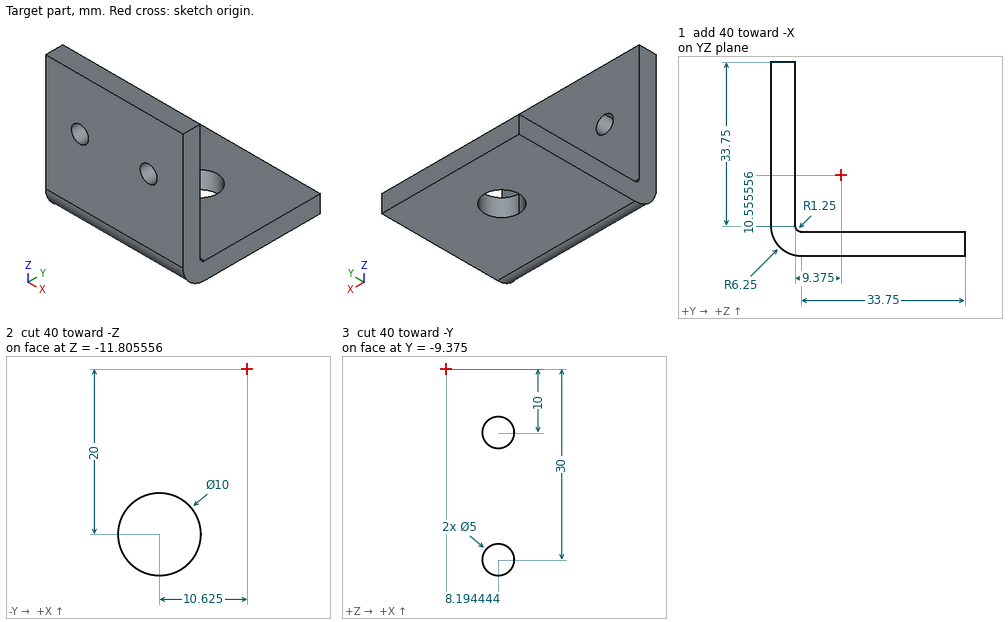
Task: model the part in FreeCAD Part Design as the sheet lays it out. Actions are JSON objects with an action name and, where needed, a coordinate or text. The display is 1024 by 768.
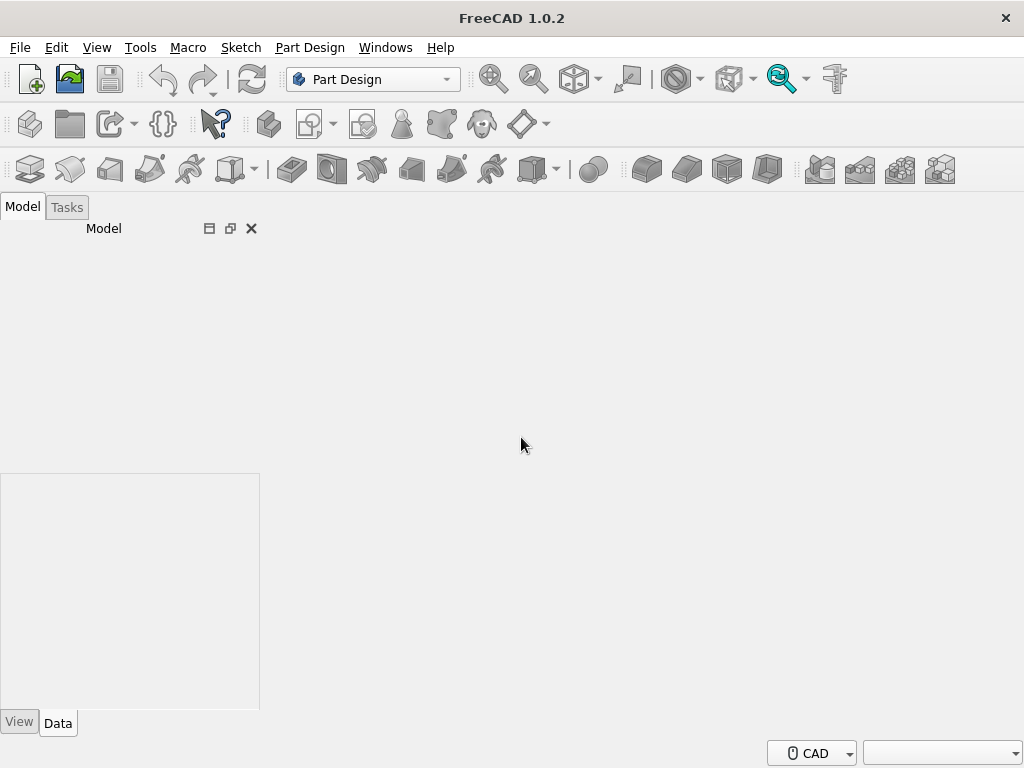
{"action": "left_click", "coordinate": [30, 80]}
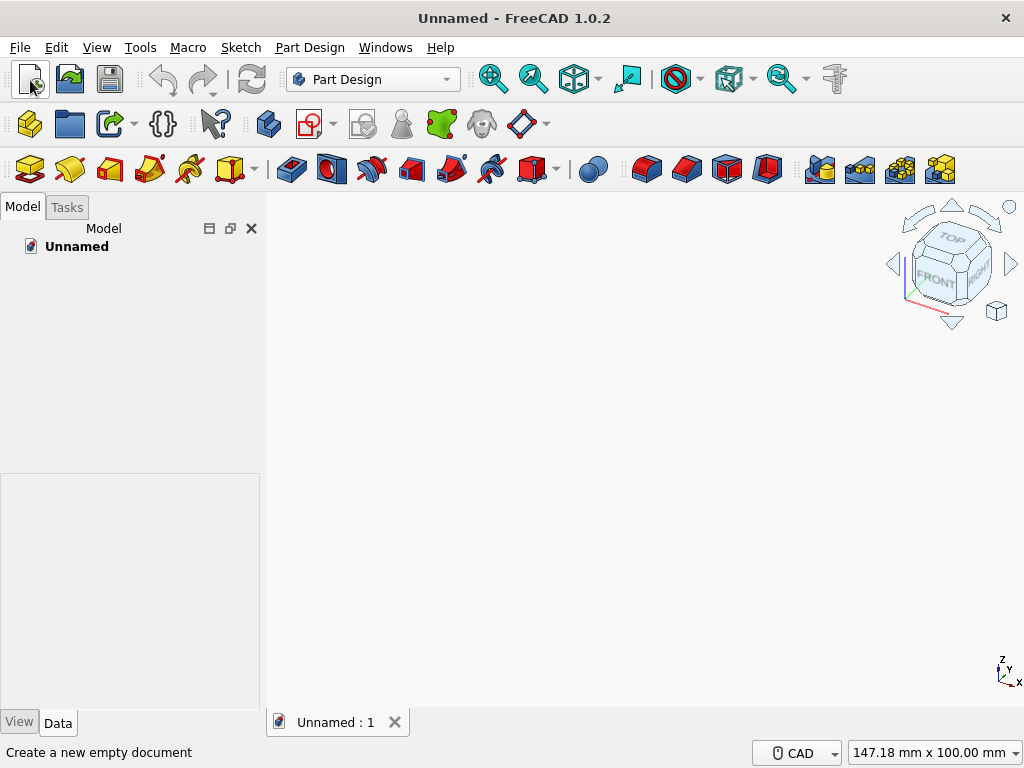
{"action": "left_click", "coordinate": [310, 124]}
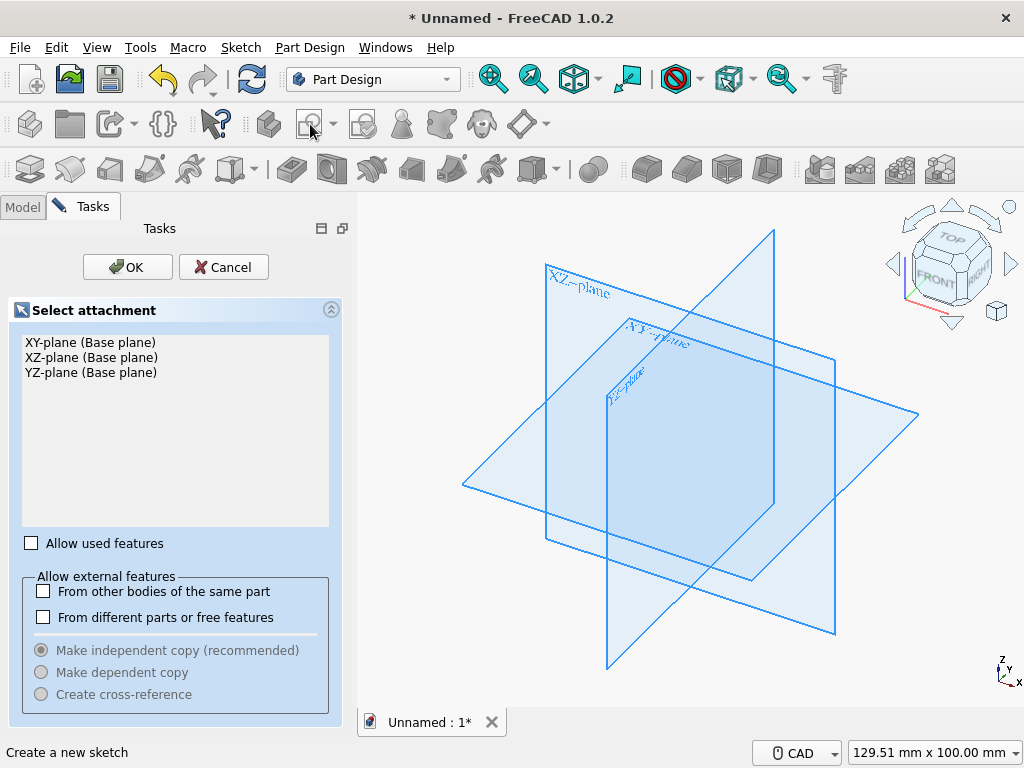
{"action": "left_click", "coordinate": [82, 372]}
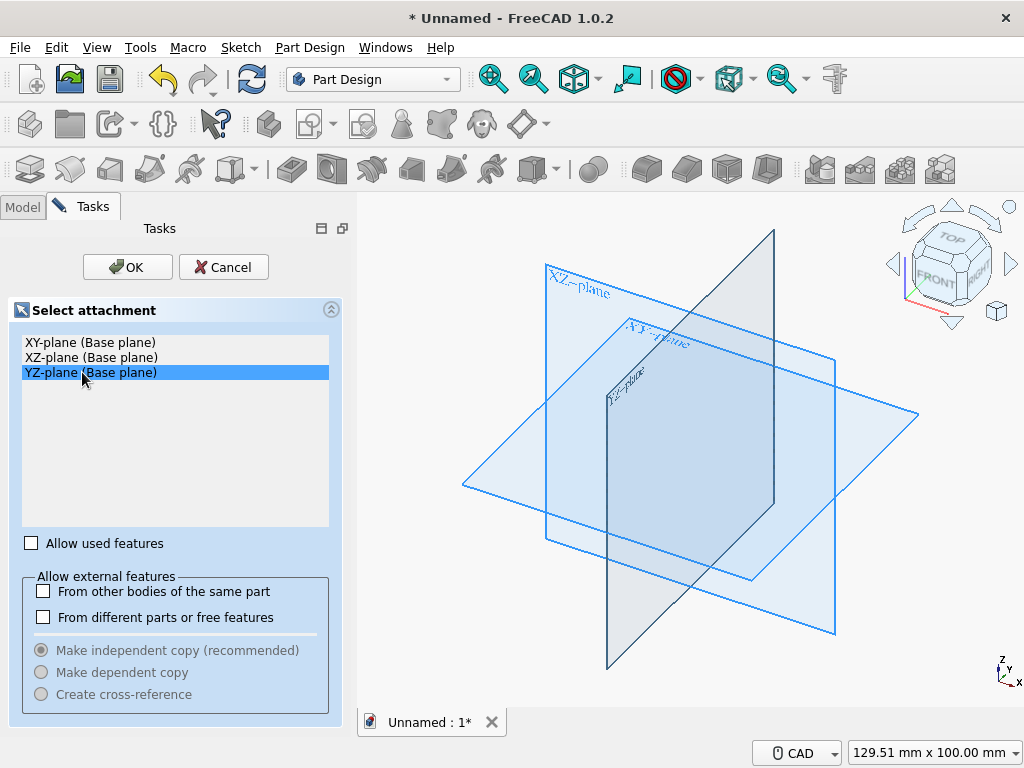
{"action": "left_click", "coordinate": [128, 267]}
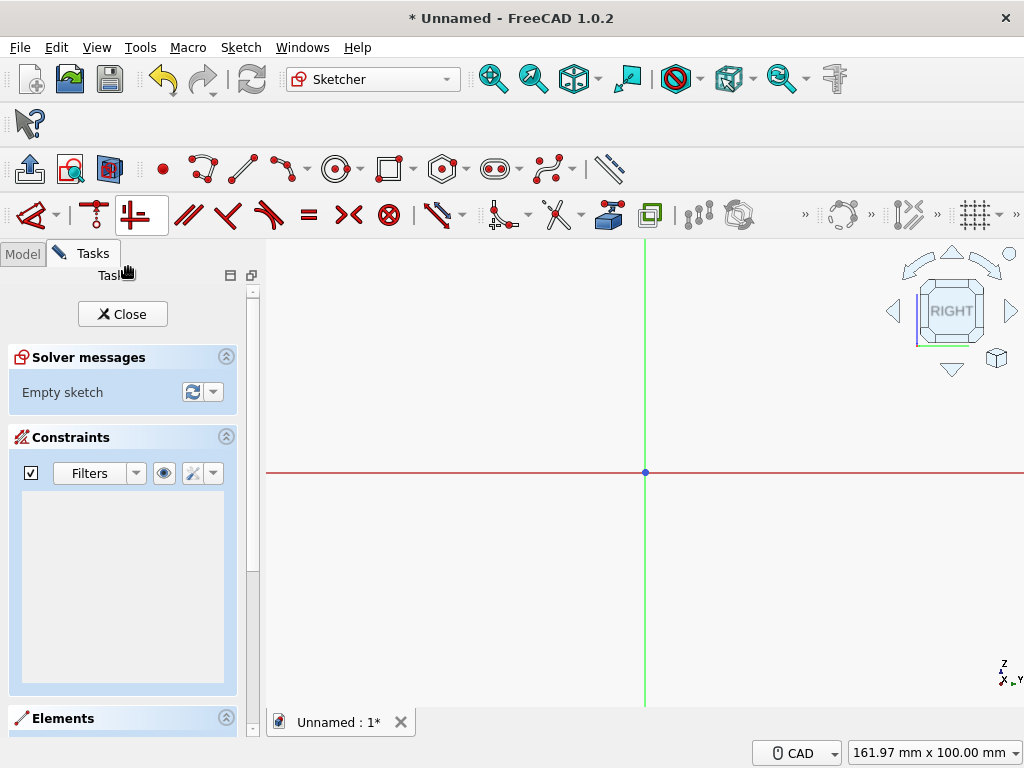
{"action": "scroll", "coordinate": [859, 428], "scroll_direction": "up", "scroll_amount": 2}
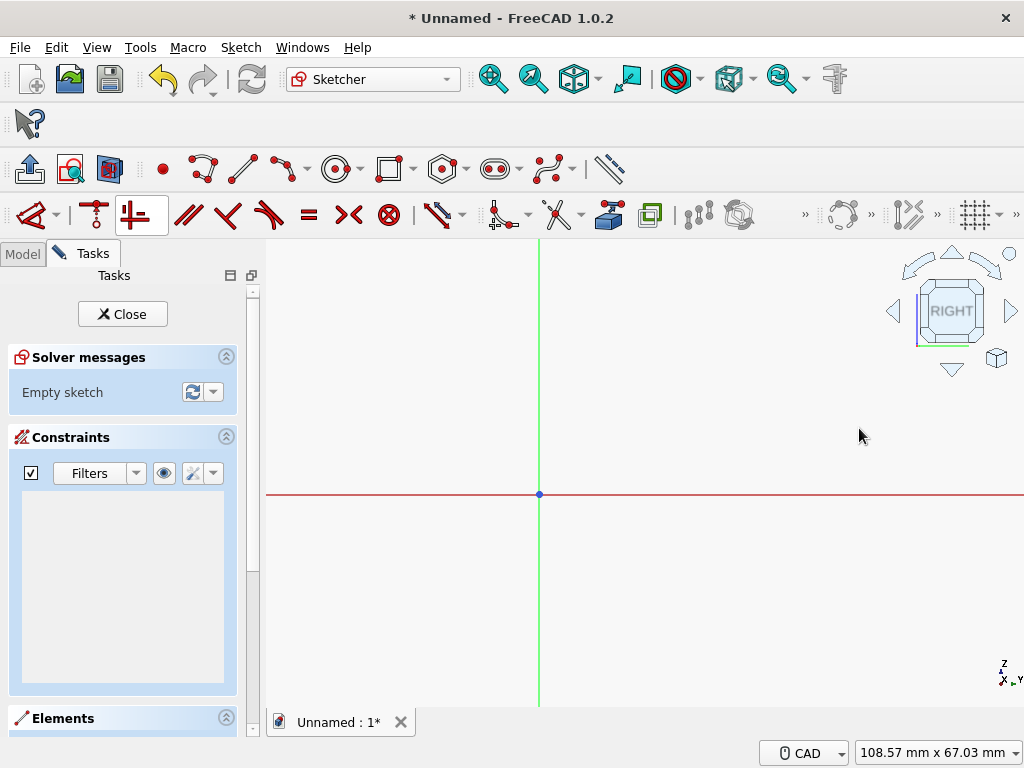
{"action": "left_click", "coordinate": [204, 170]}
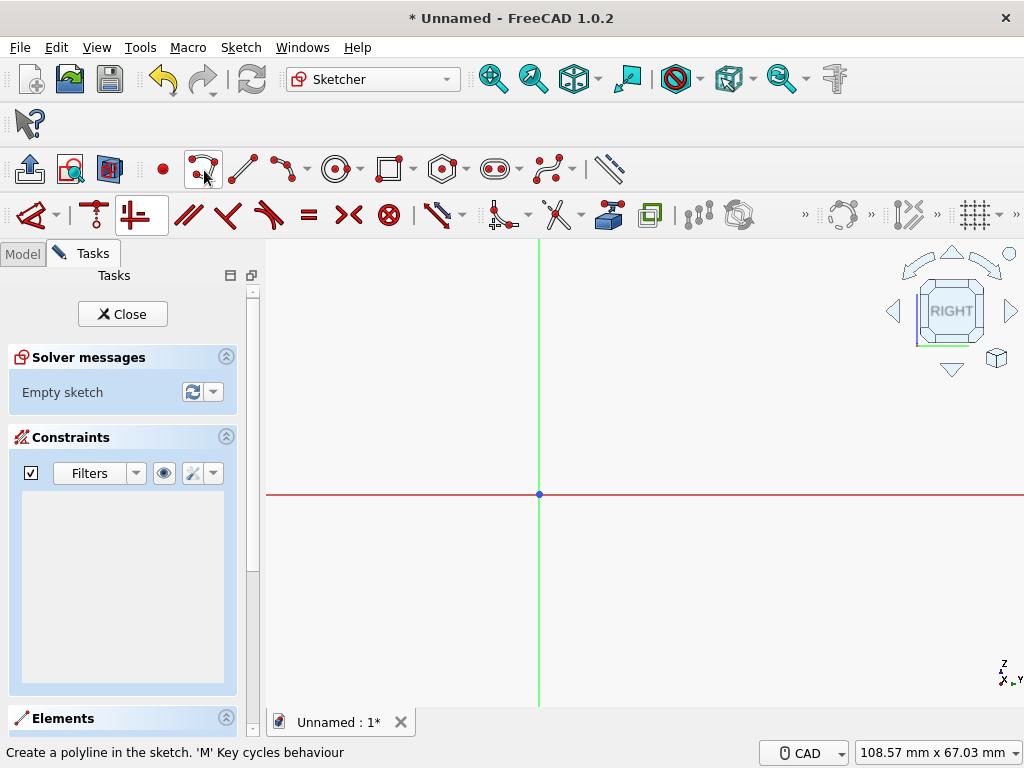
{"action": "left_click", "coordinate": [474, 569]}
{"action": "left_click", "coordinate": [474, 333]}
{"action": "left_click", "coordinate": [439, 333]}
{"action": "left_click", "coordinate": [439, 569]}
{"action": "right_click", "coordinate": [439, 569]}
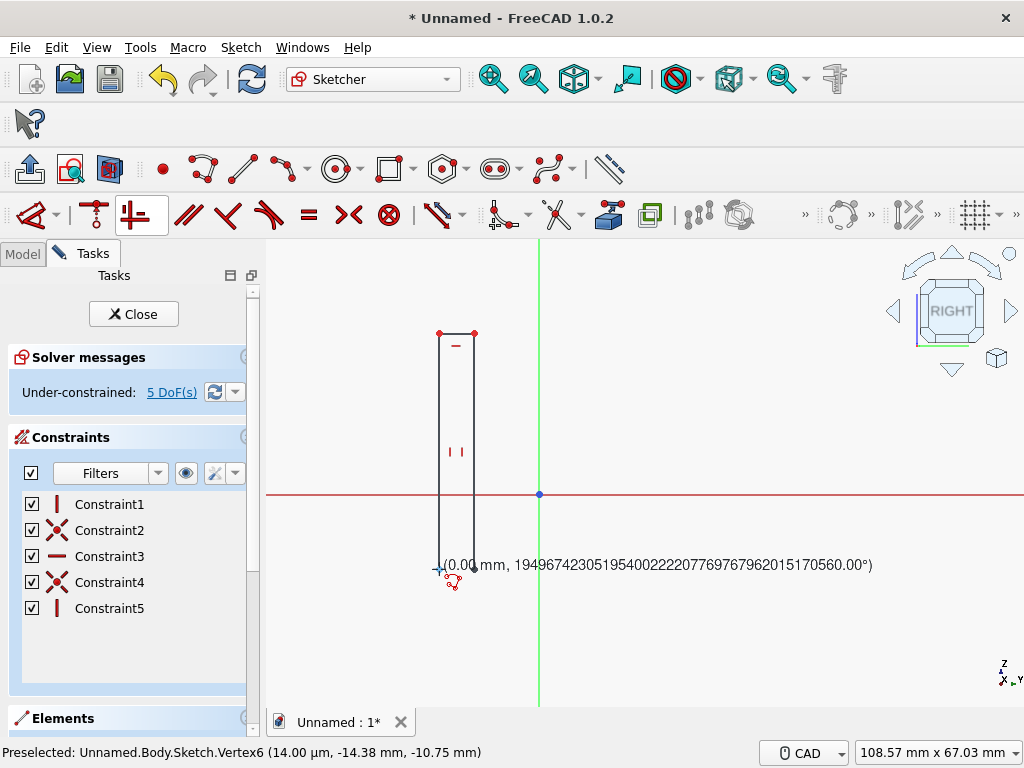
{"action": "left_click", "coordinate": [483, 612]}
{"action": "left_click", "coordinate": [718, 612]}
{"action": "left_click", "coordinate": [718, 577]}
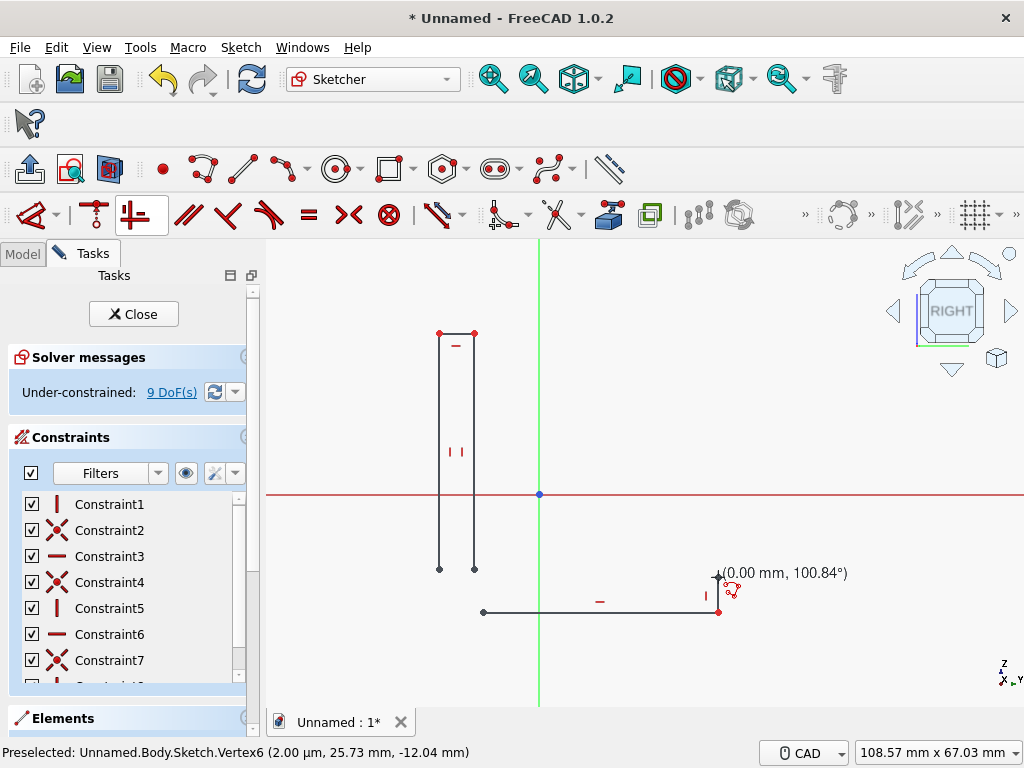
{"action": "scroll", "coordinate": [483, 577], "scroll_direction": "up", "scroll_amount": 2}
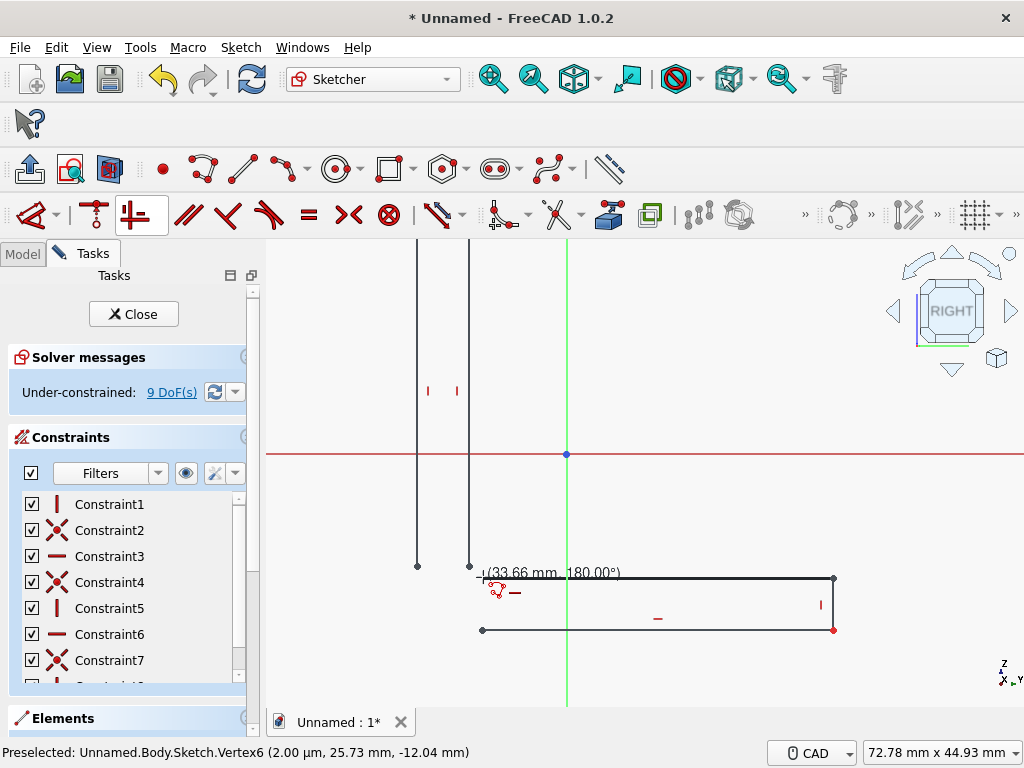
{"action": "left_click", "coordinate": [482, 577]}
{"action": "right_click", "coordinate": [482, 577]}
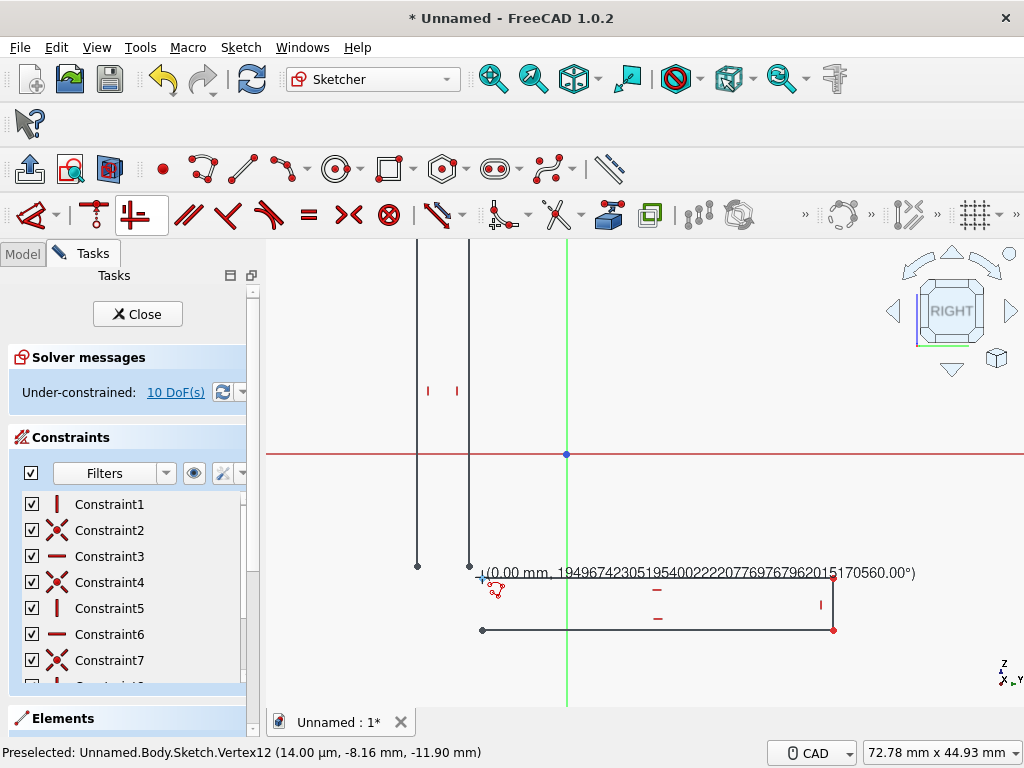
{"action": "key", "text": "g 3 a"}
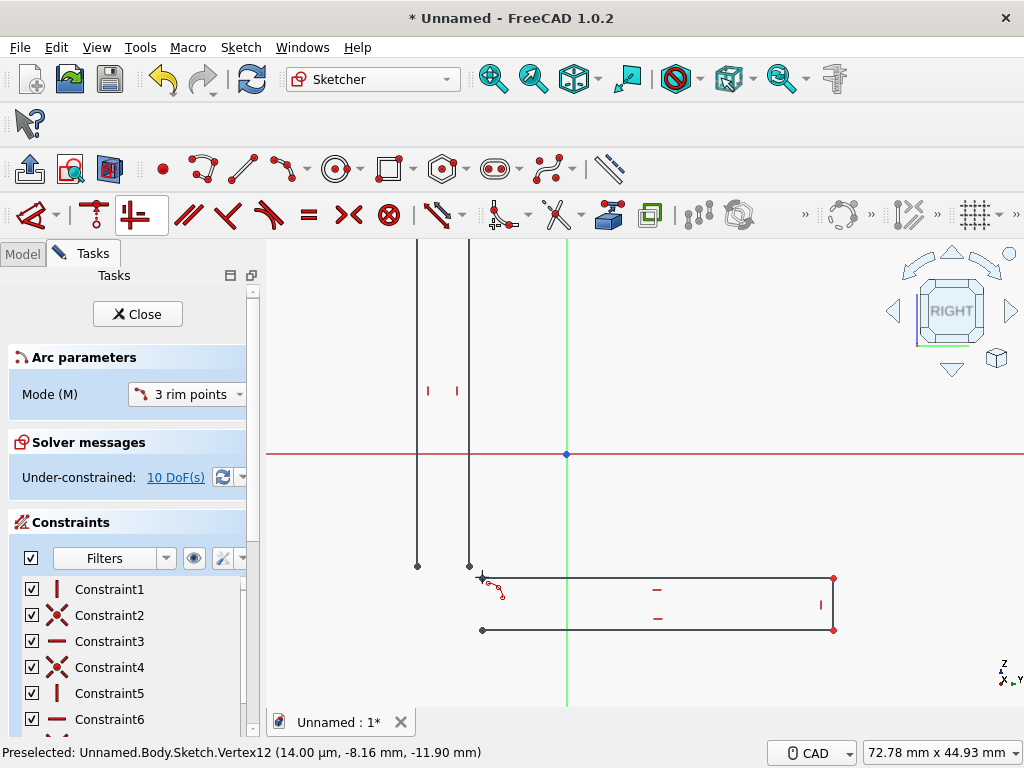
{"action": "left_click", "coordinate": [417, 566]}
{"action": "left_click", "coordinate": [483, 630]}
{"action": "left_click", "coordinate": [436, 610]}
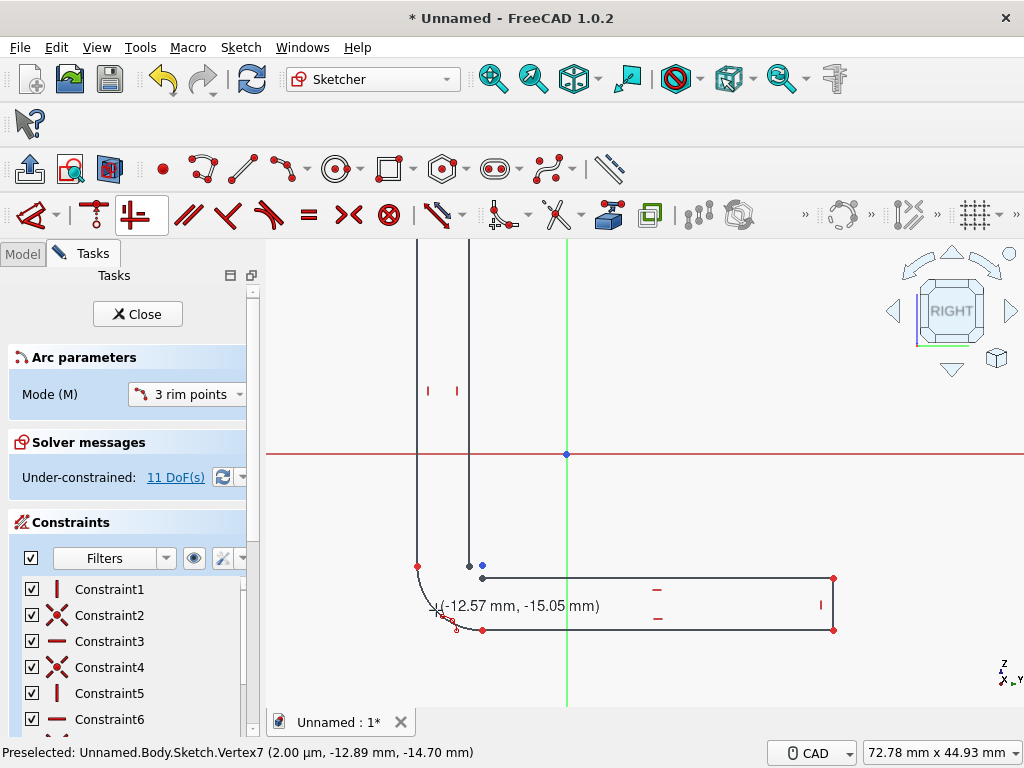
{"action": "left_click", "coordinate": [482, 578]}
{"action": "left_click", "coordinate": [469, 566]}